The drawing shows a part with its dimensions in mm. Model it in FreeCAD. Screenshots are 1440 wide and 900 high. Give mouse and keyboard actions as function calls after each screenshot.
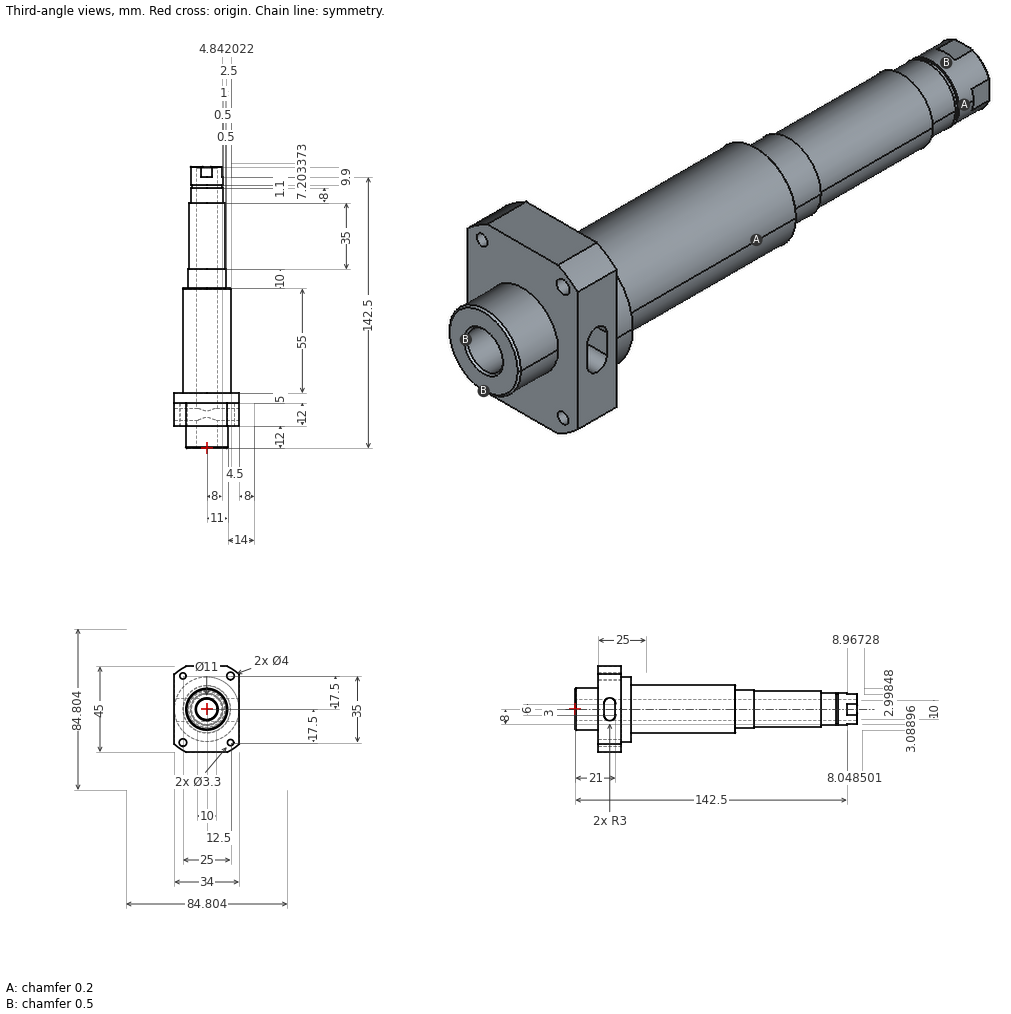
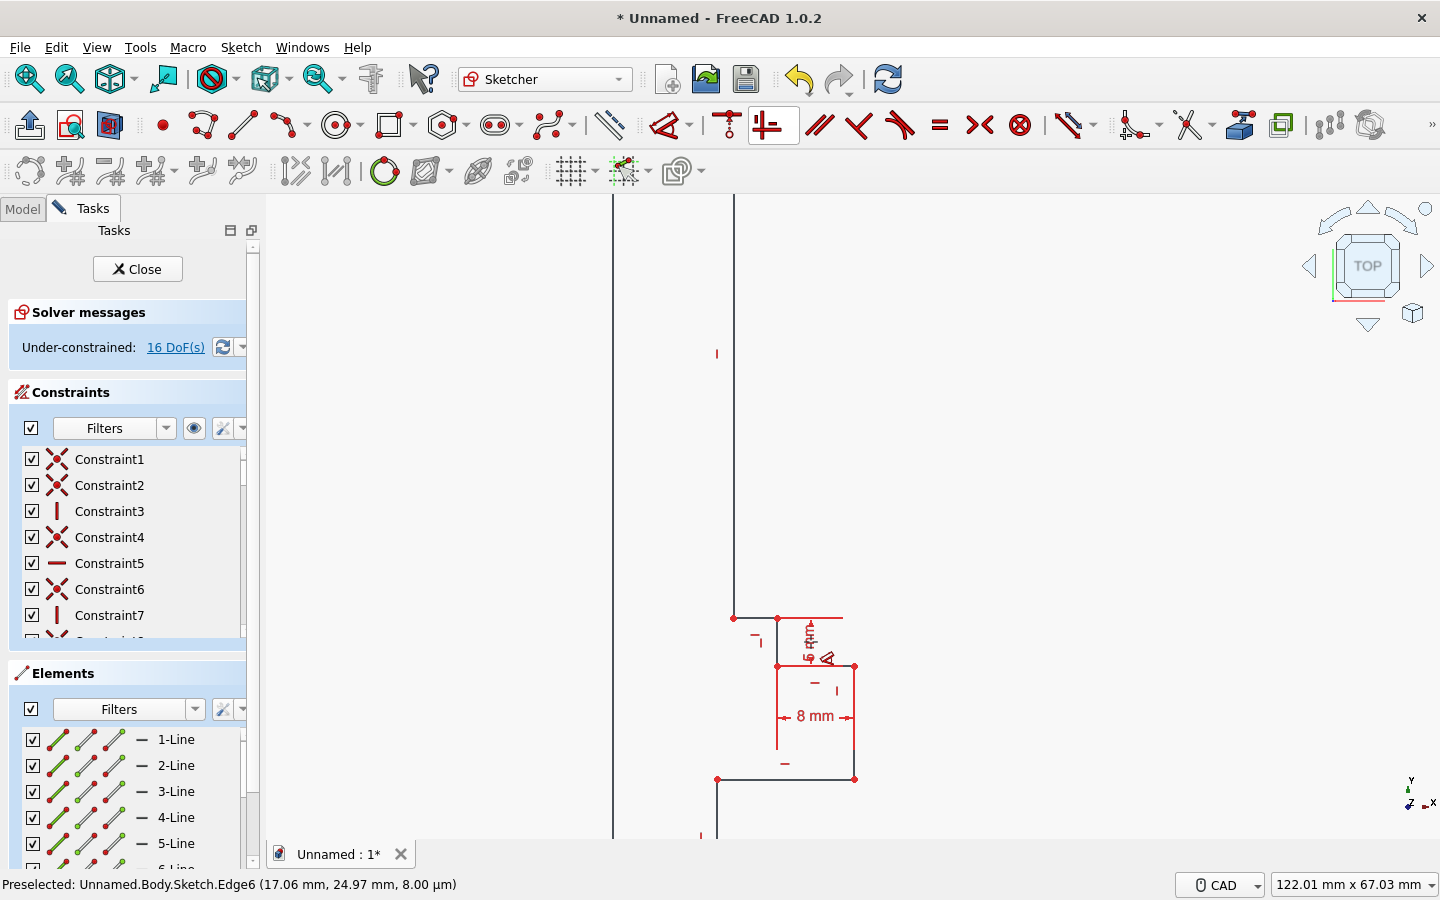
scroll(807, 661, down, 6)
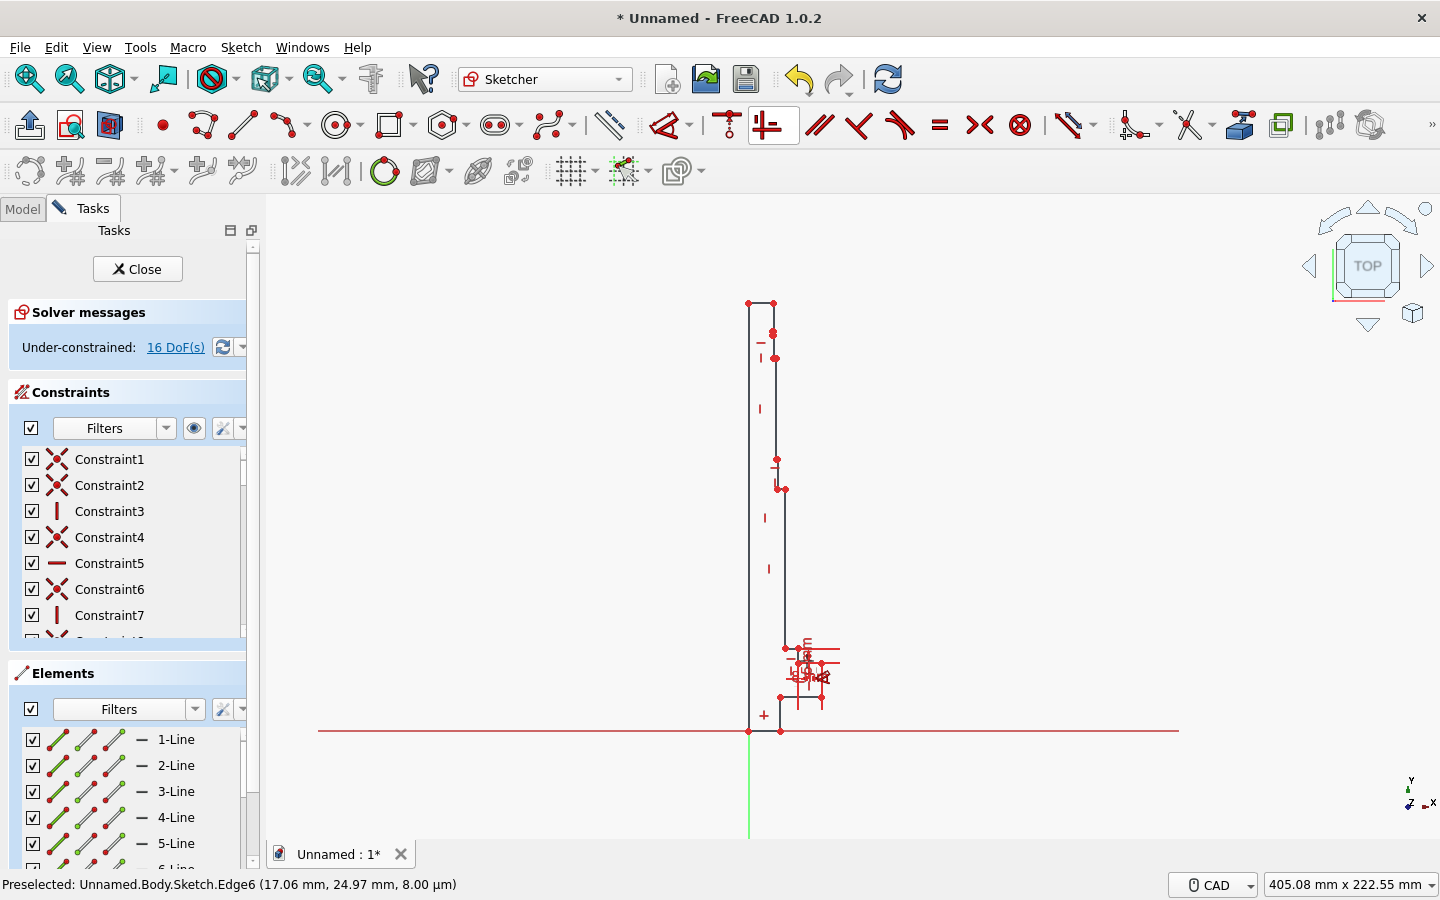
scroll(775, 358, up, 14)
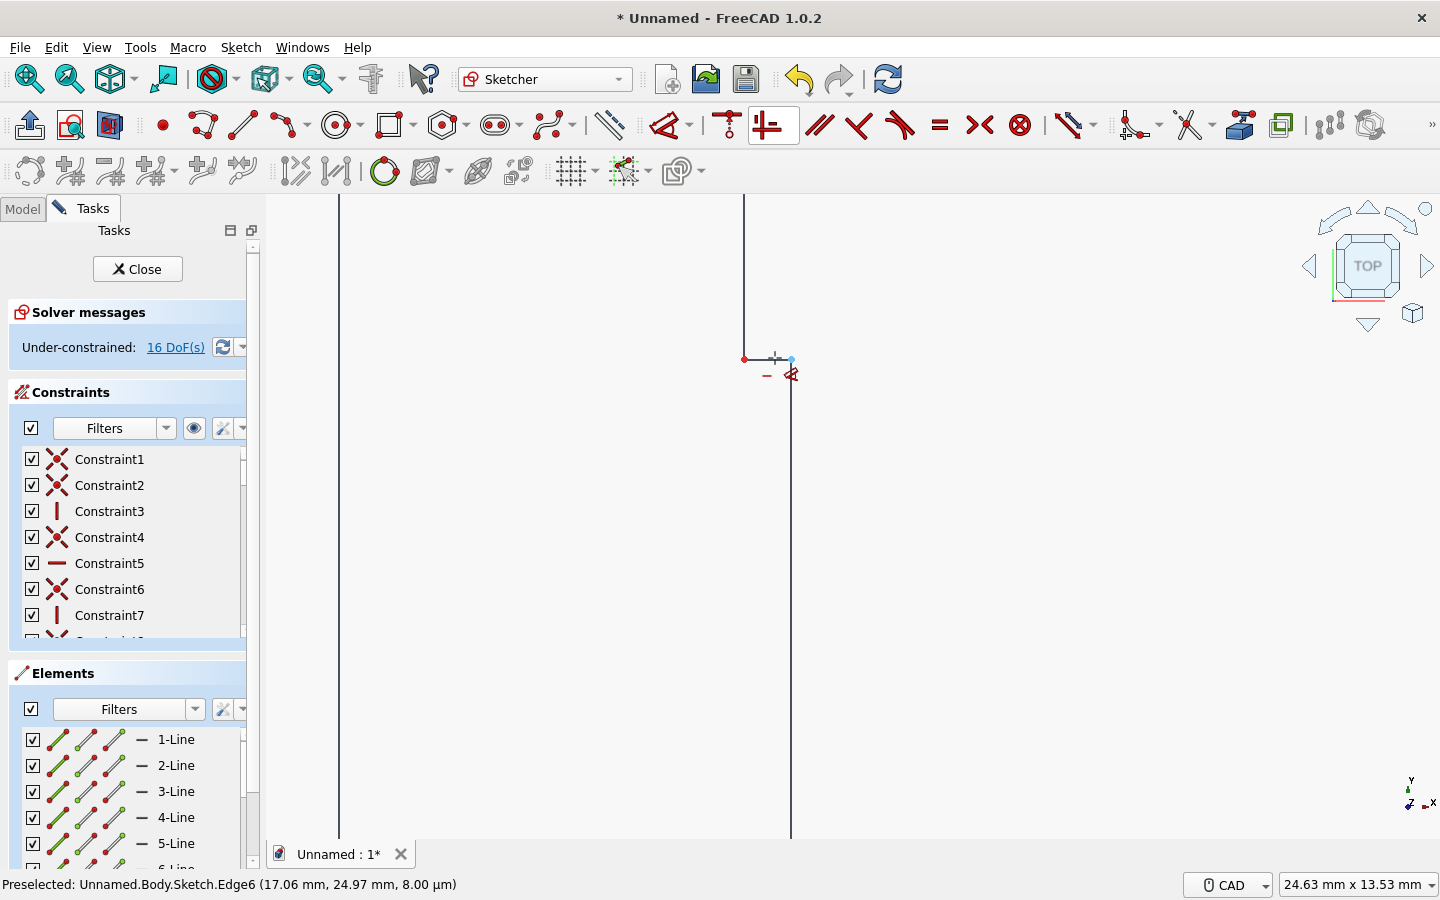
click(768, 360)
click(768, 326)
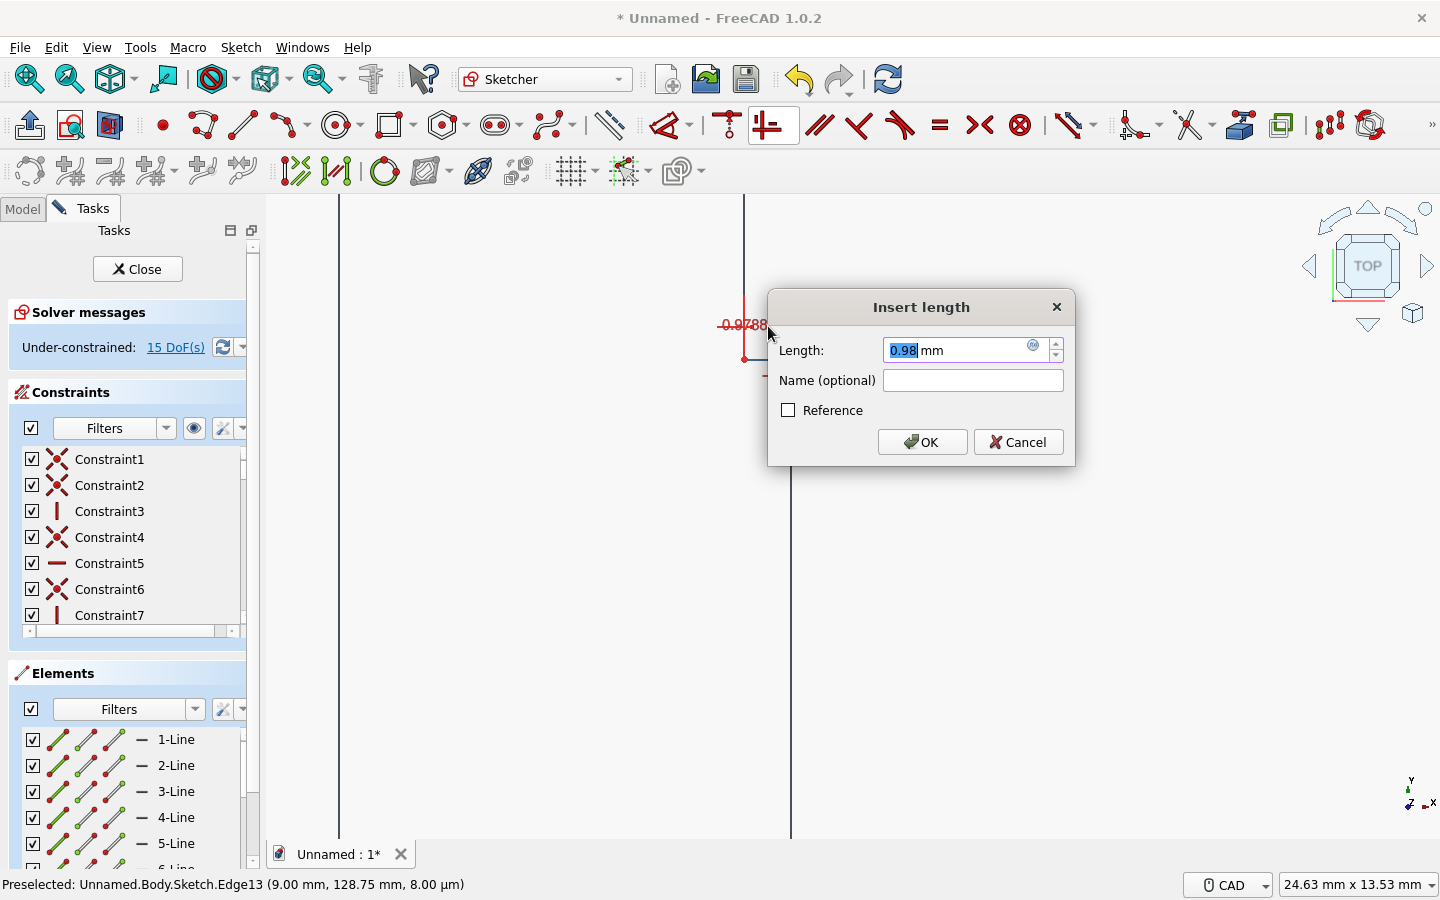
text(1)
key(Return)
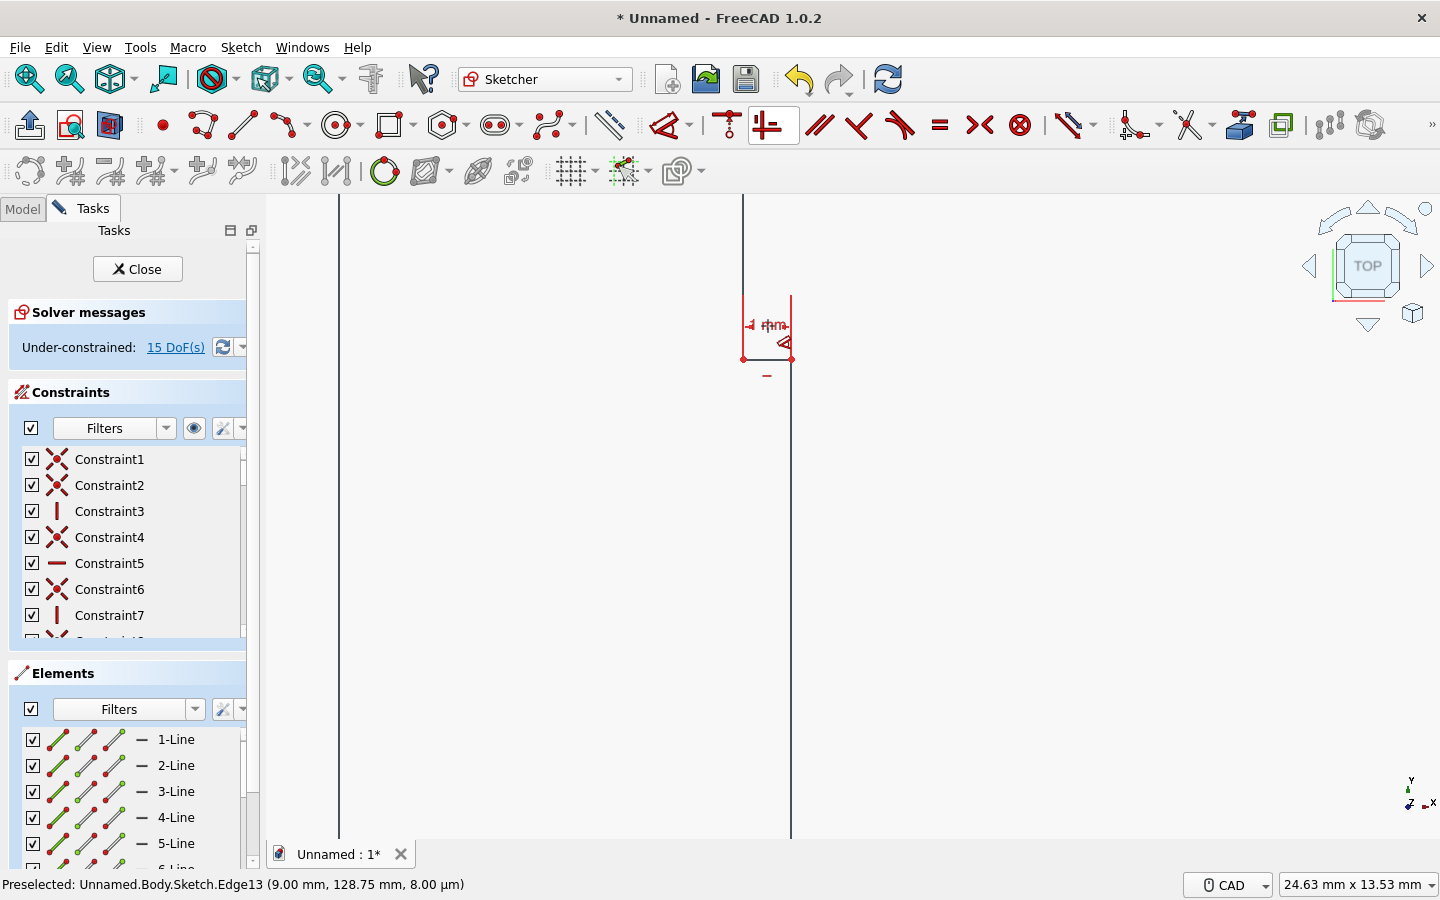
scroll(775, 358, down, 14)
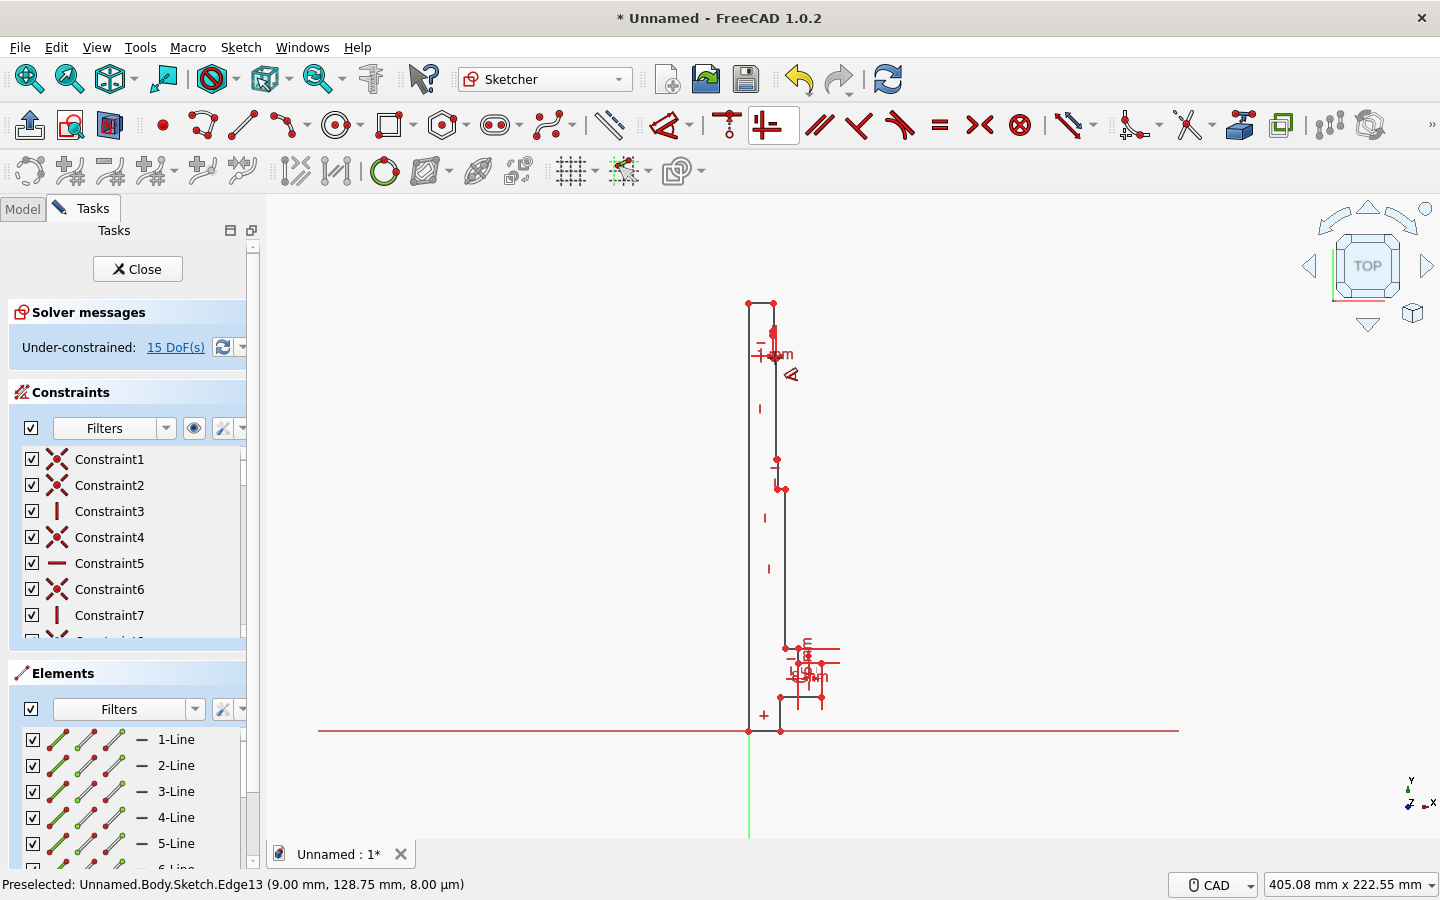
scroll(773, 351, up, 4)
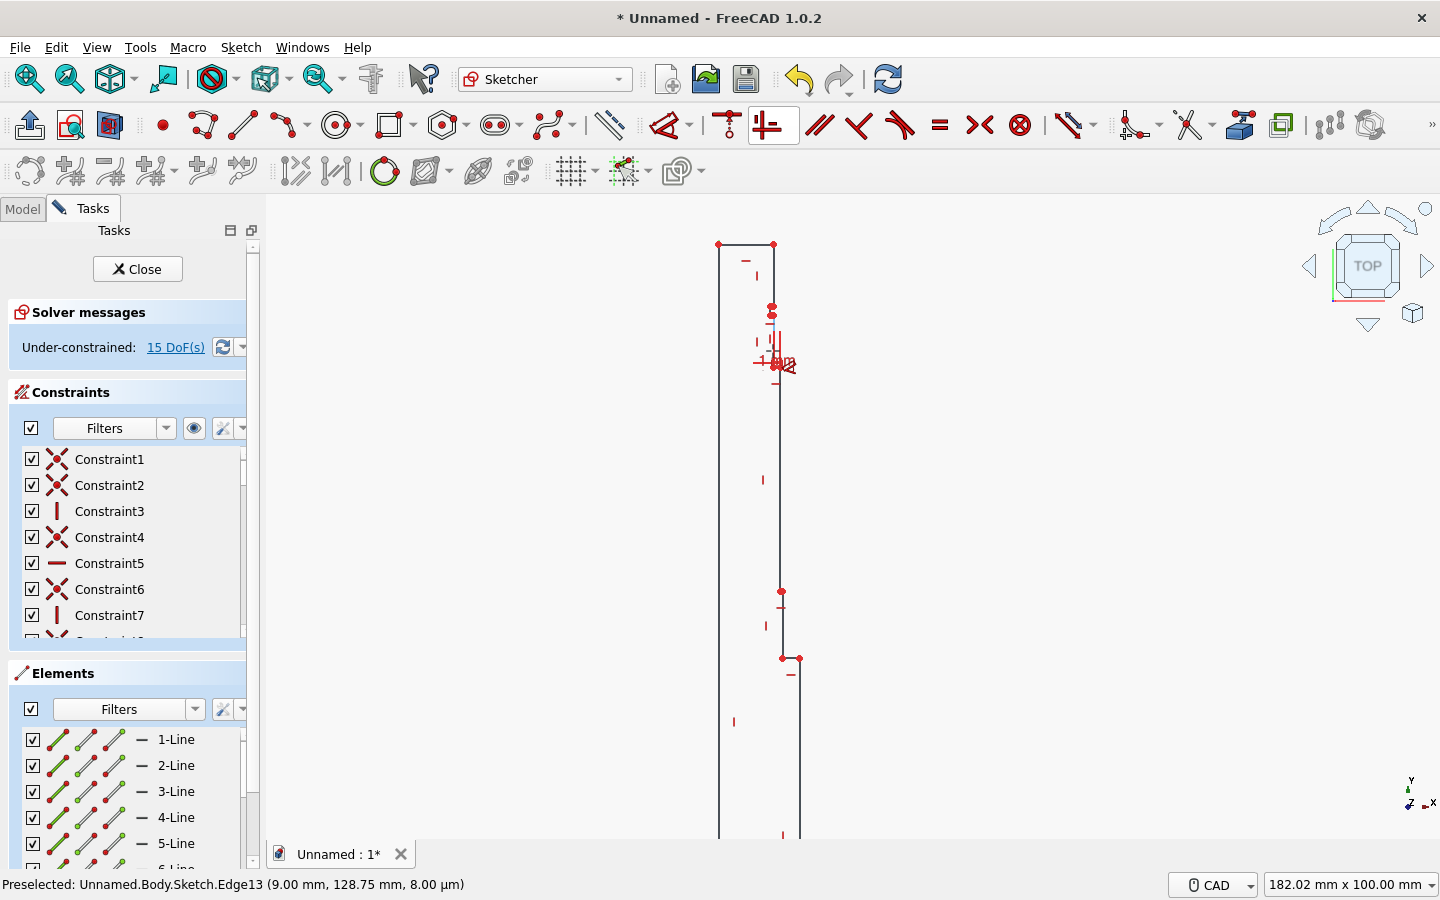
click(774, 352)
click(740, 341)